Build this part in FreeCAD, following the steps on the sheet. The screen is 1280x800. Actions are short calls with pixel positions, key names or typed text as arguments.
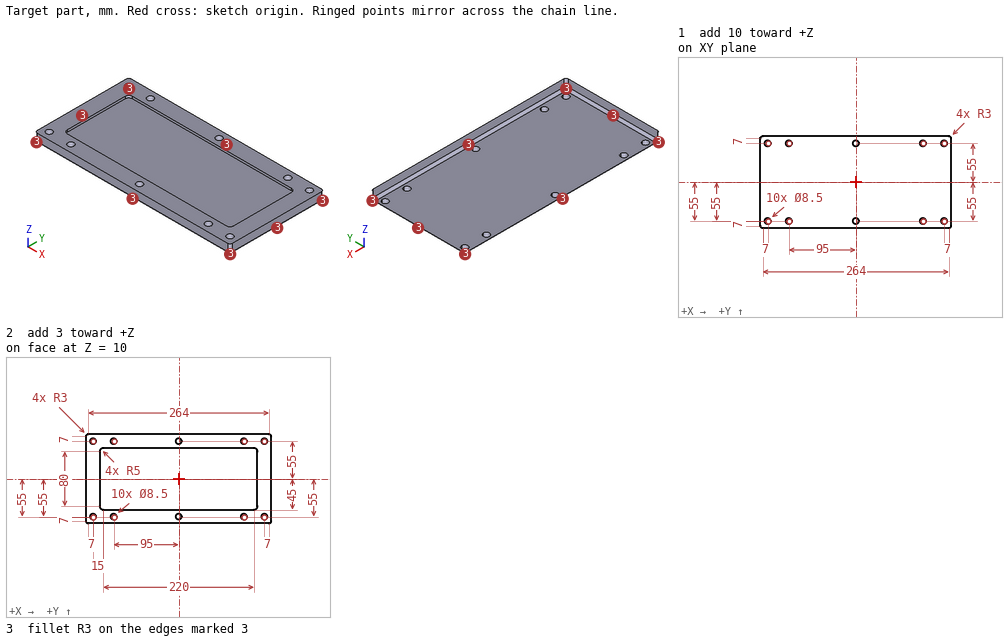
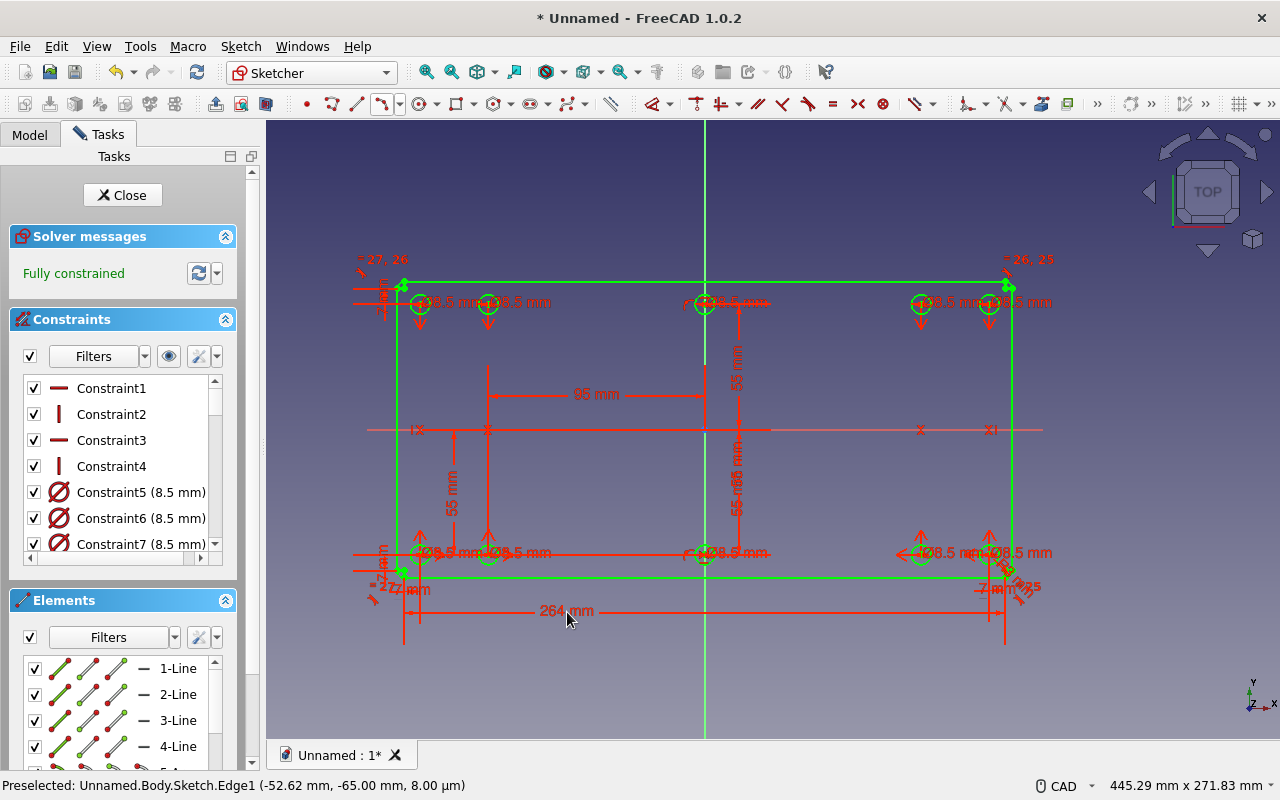
click(123, 195)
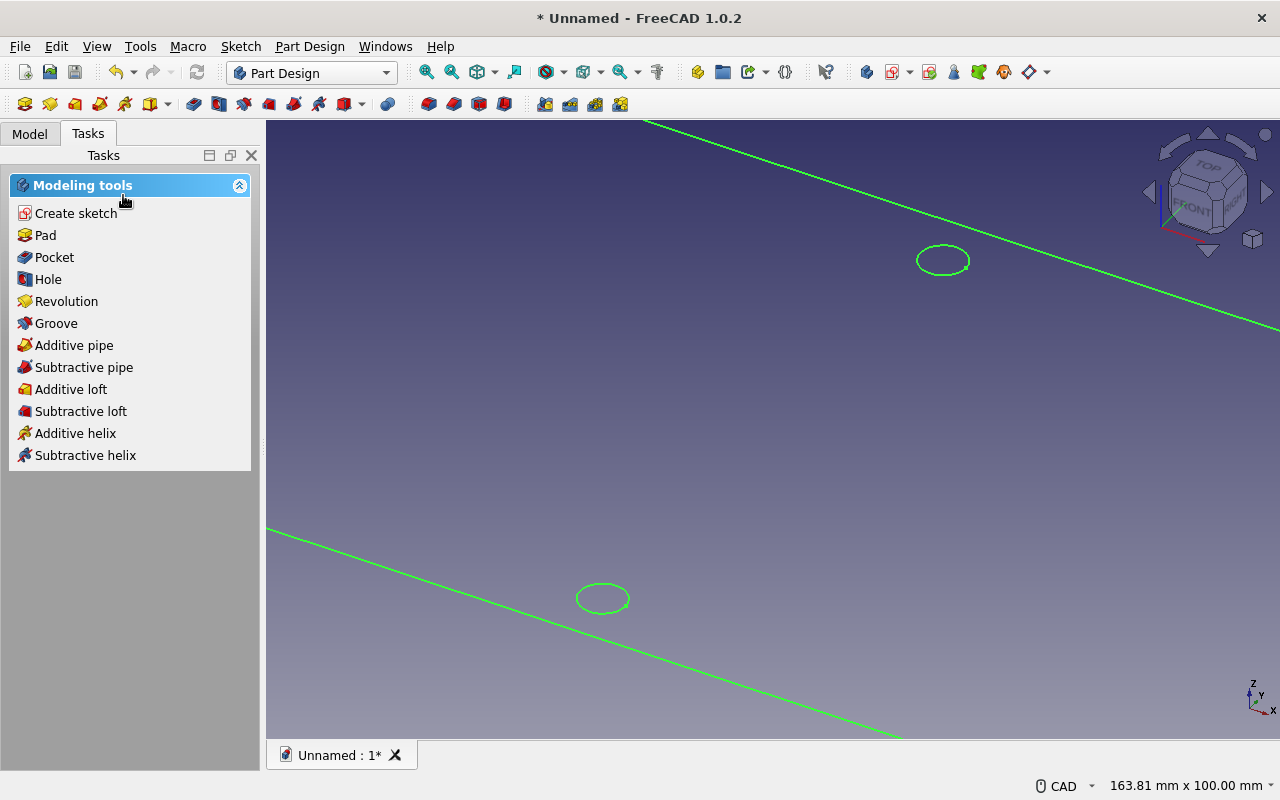
click(25, 104)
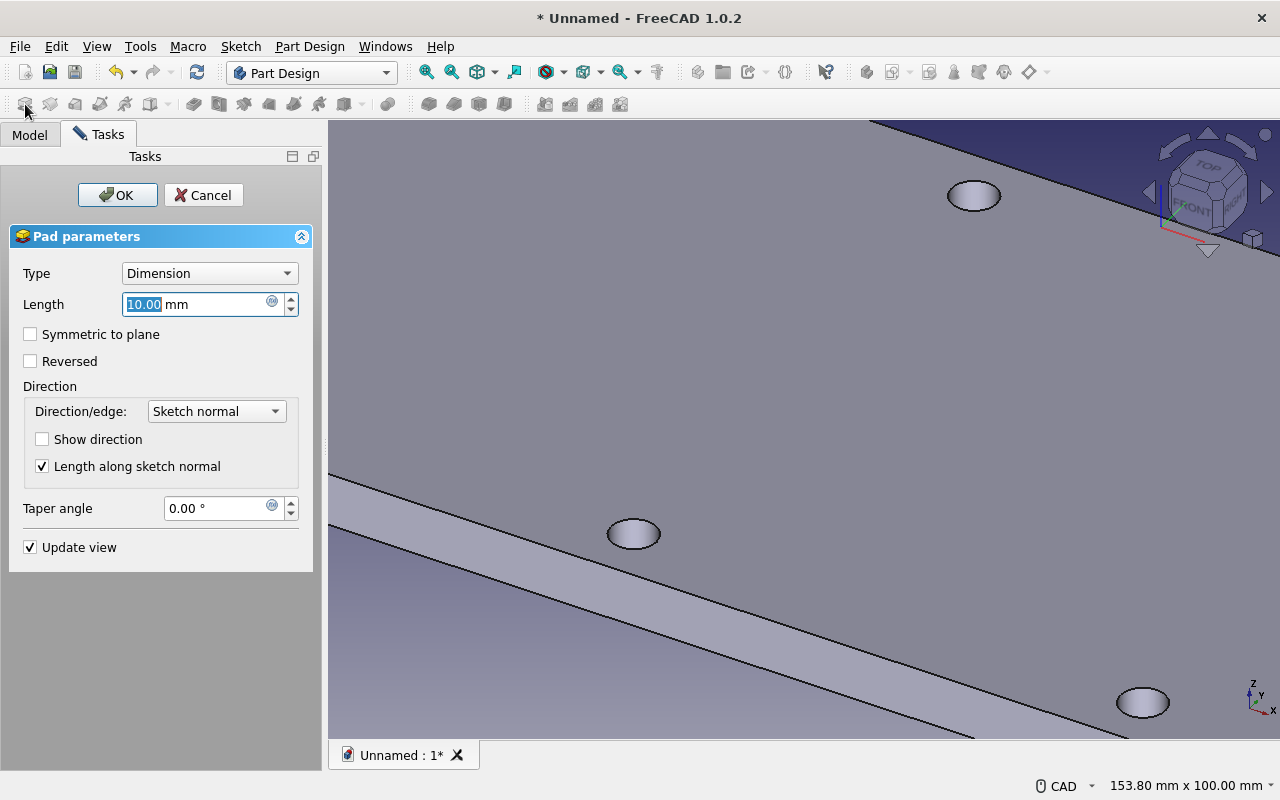
text(10)
key(Tab)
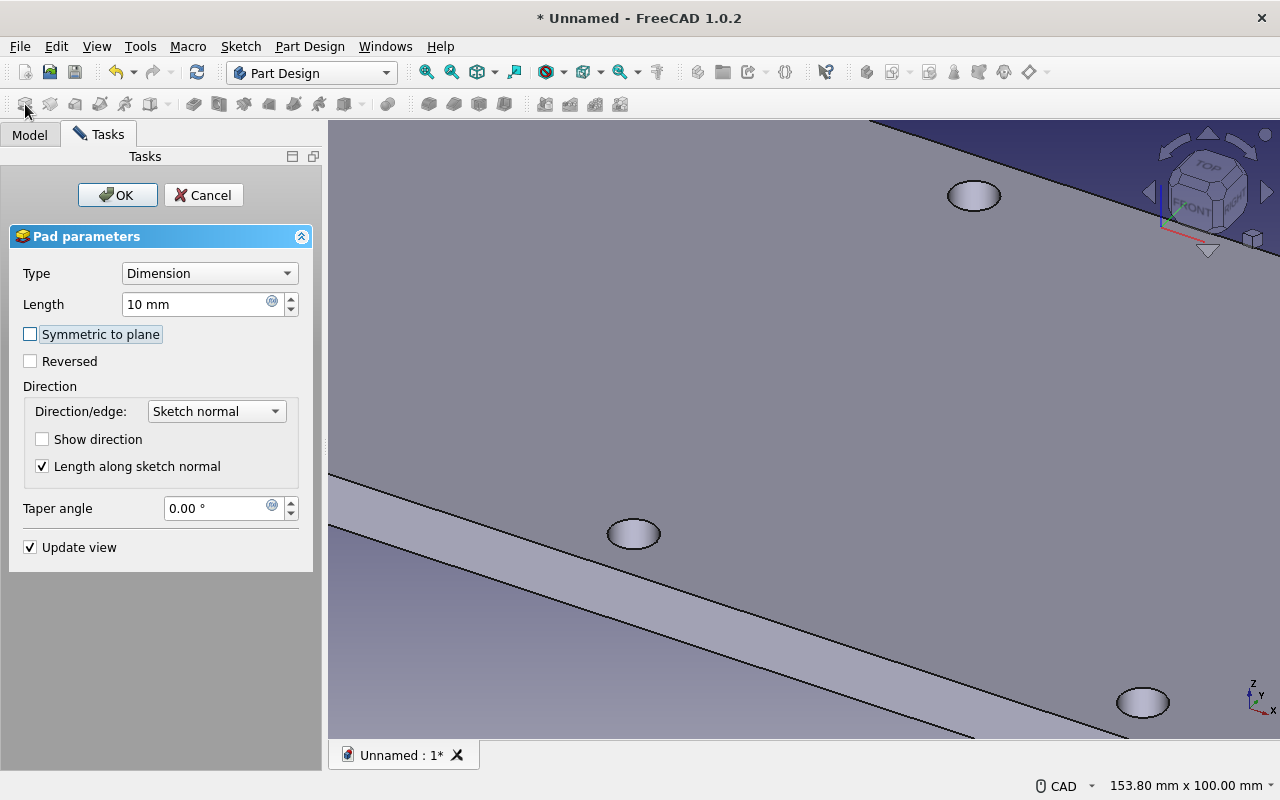
click(118, 195)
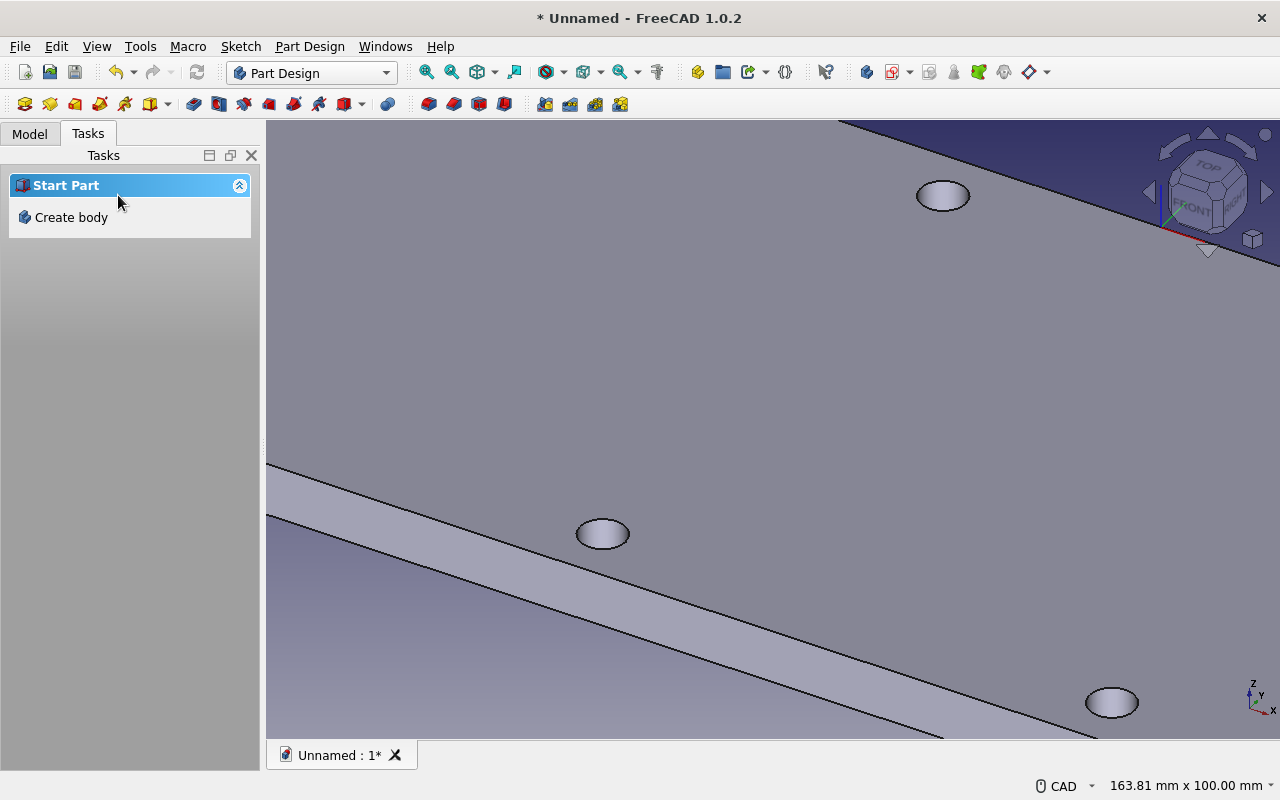
click(427, 72)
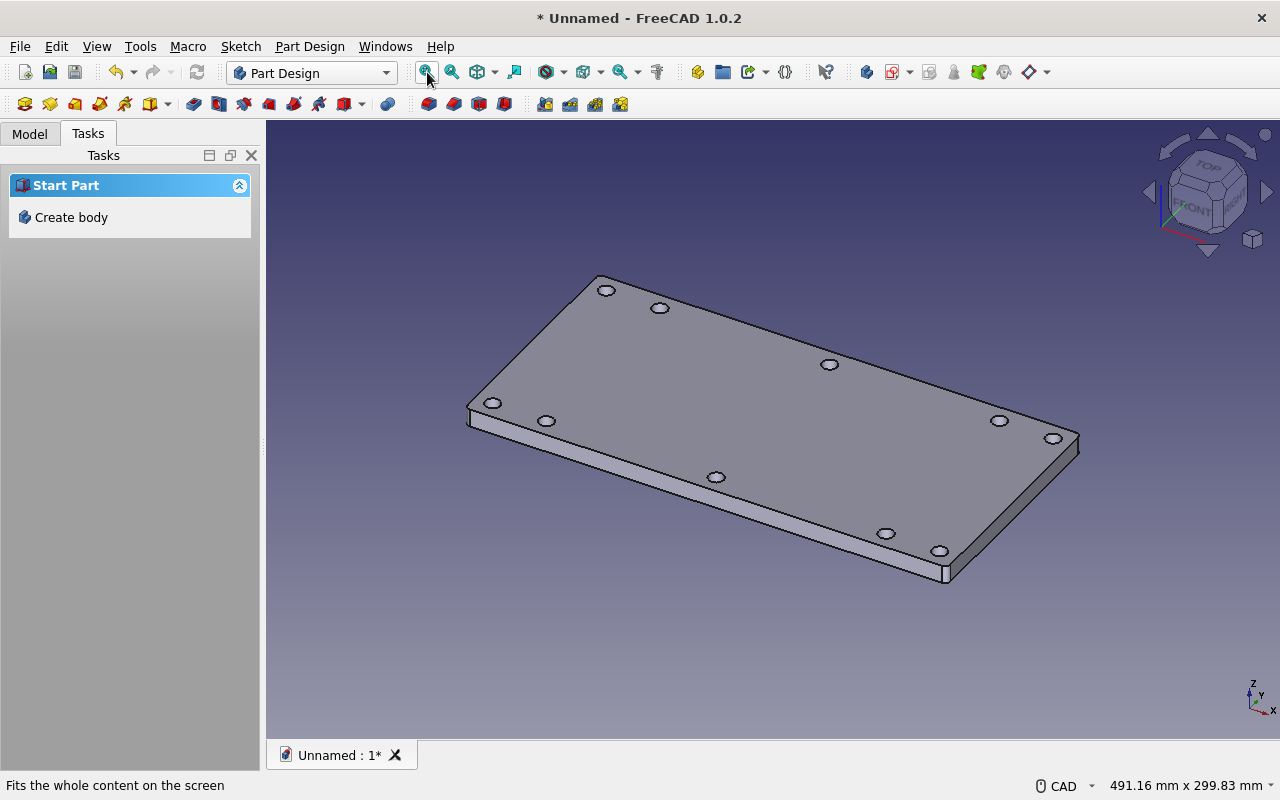
click(704, 397)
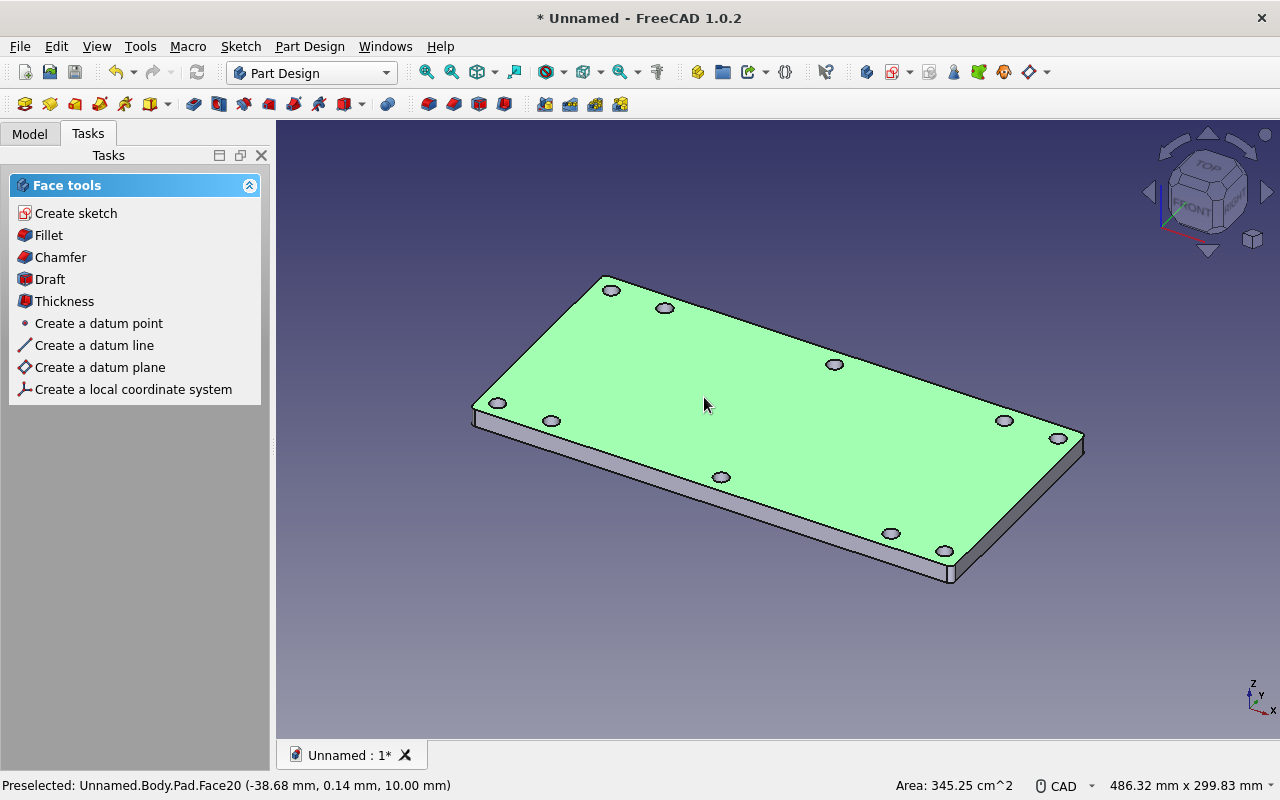
click(892, 72)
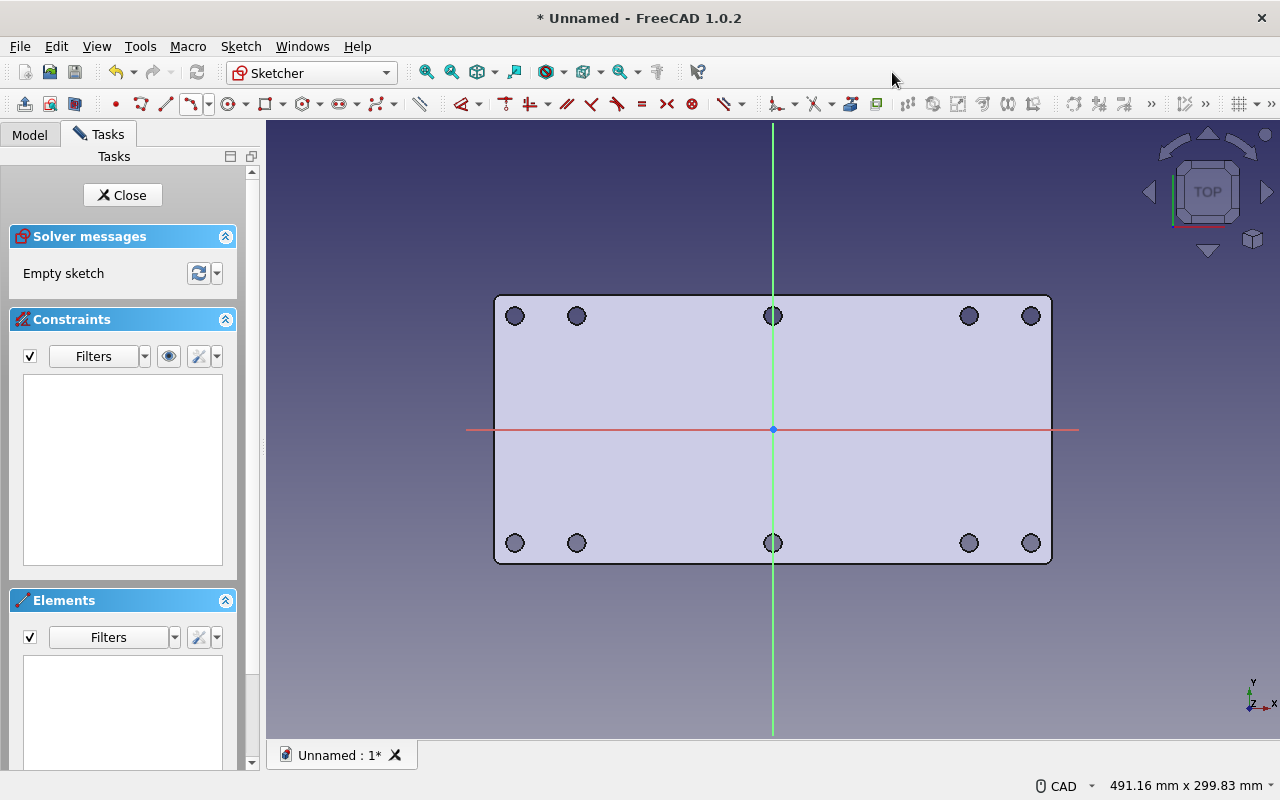
click(166, 104)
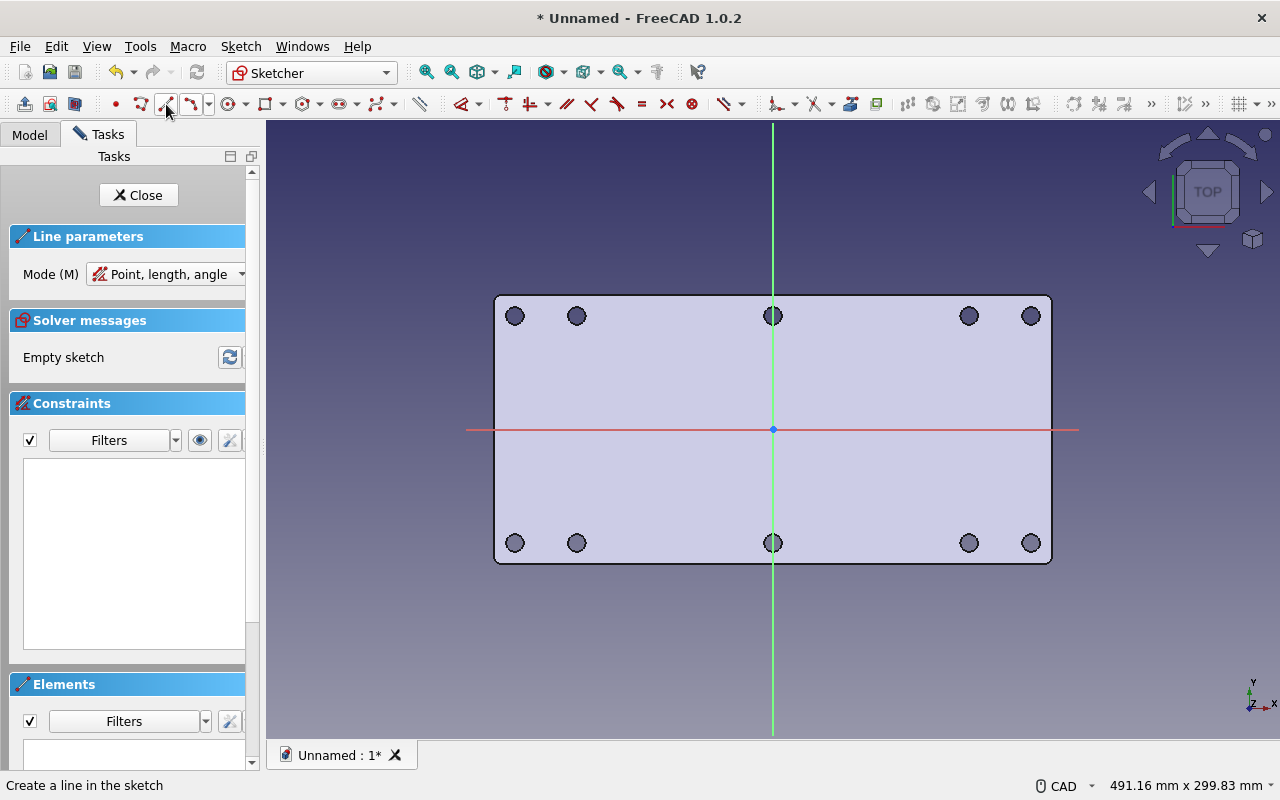
click(1046, 295)
click(500, 295)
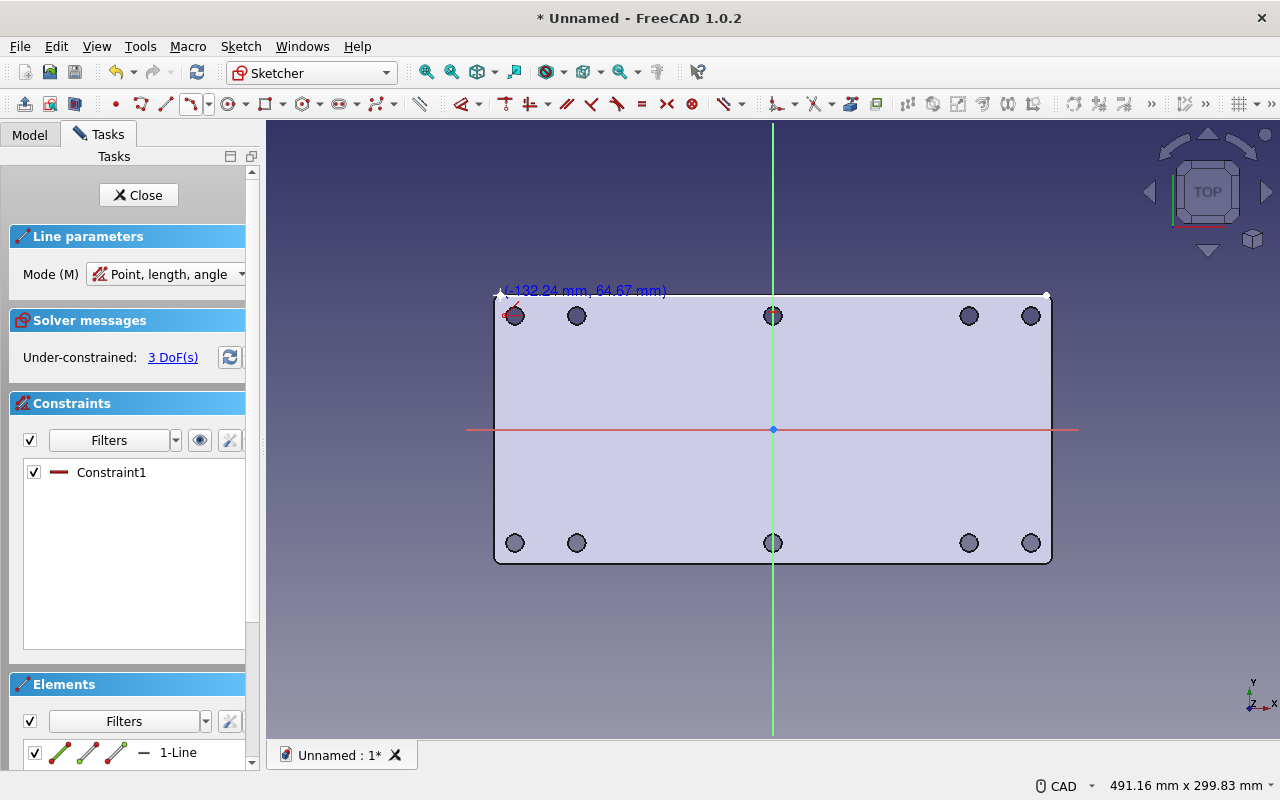
scroll(494, 302, up, 3)